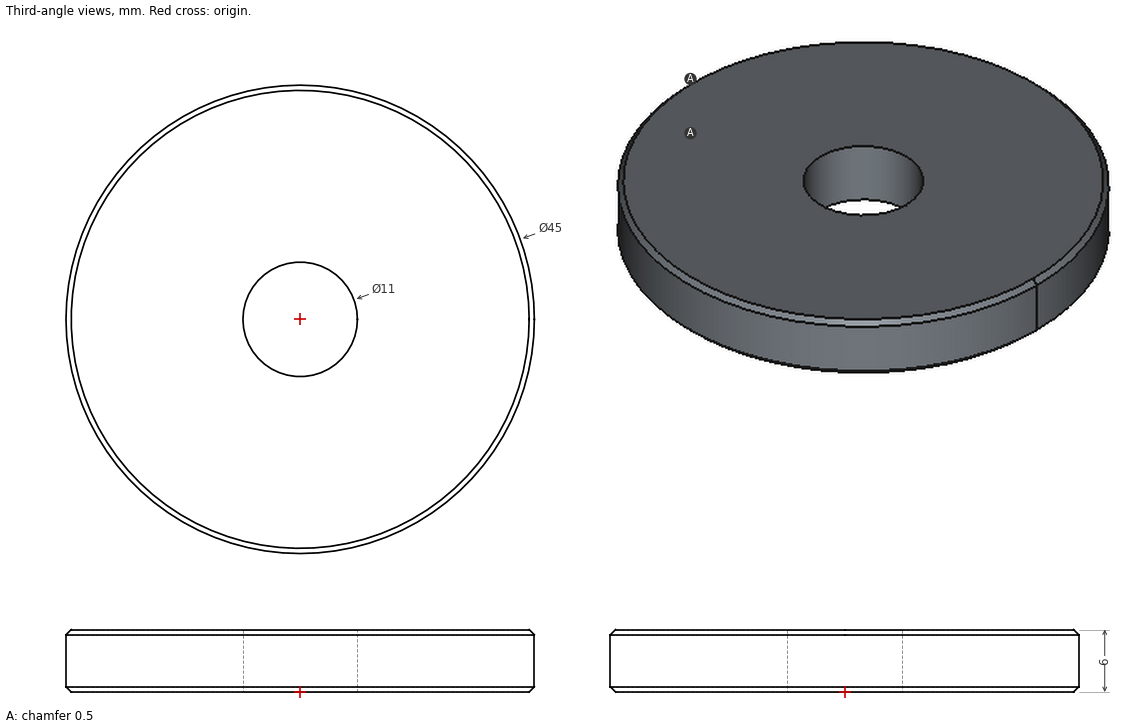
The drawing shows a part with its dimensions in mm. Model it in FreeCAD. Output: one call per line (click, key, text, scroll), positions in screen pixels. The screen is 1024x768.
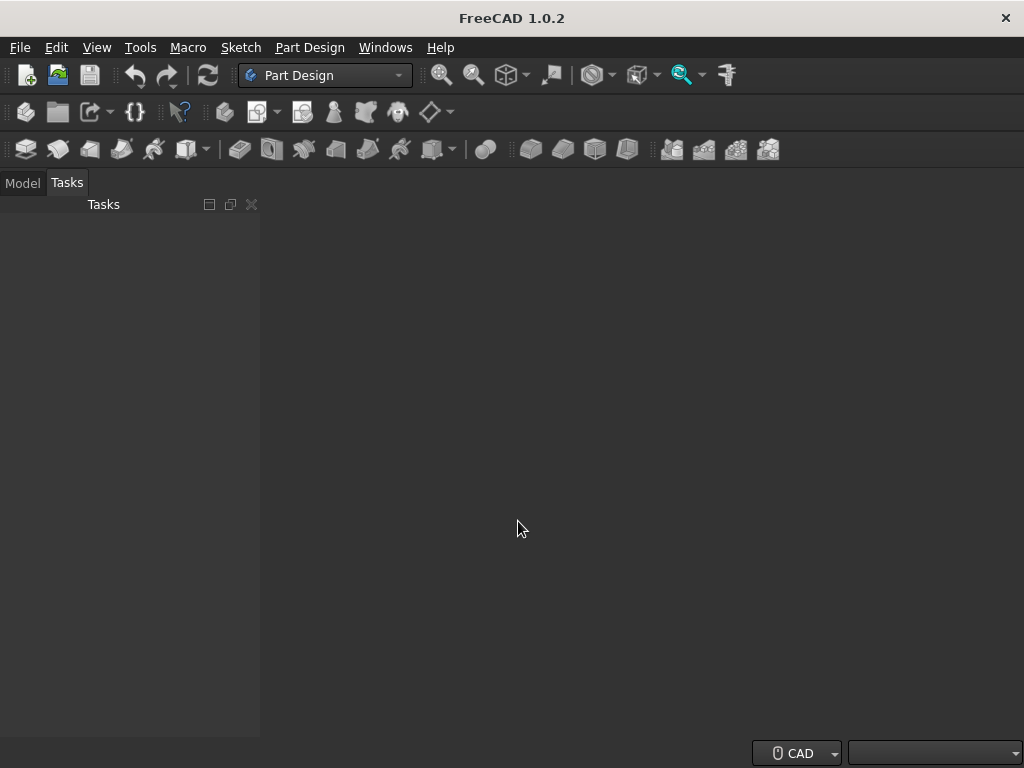
click(26, 76)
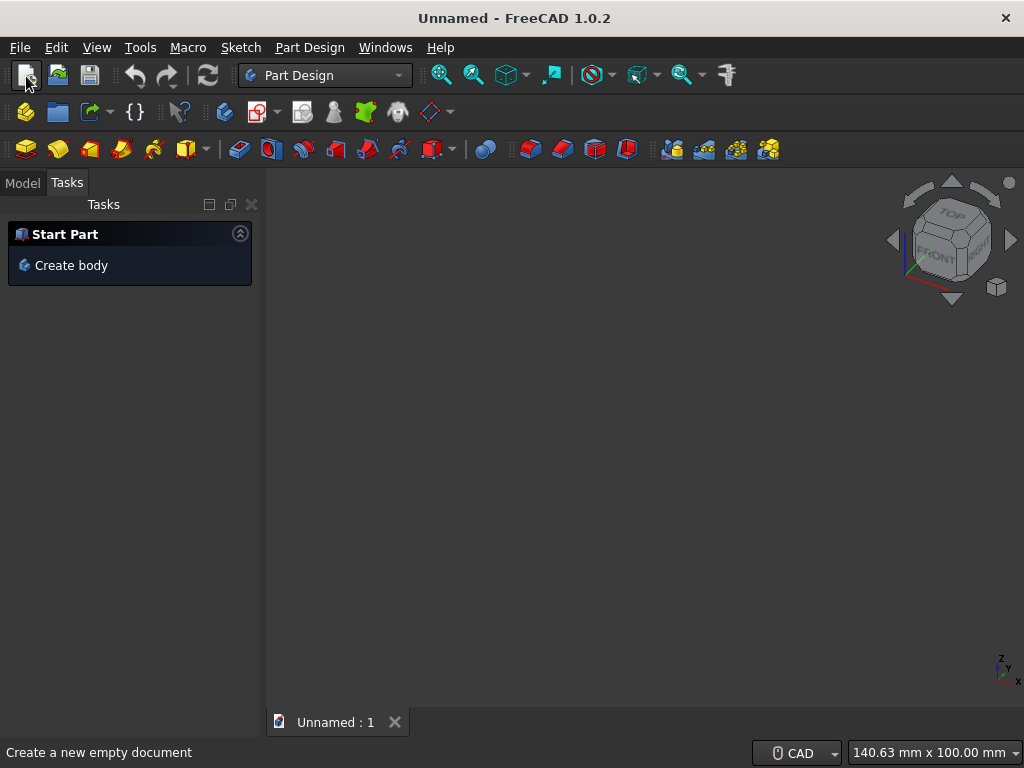
click(258, 112)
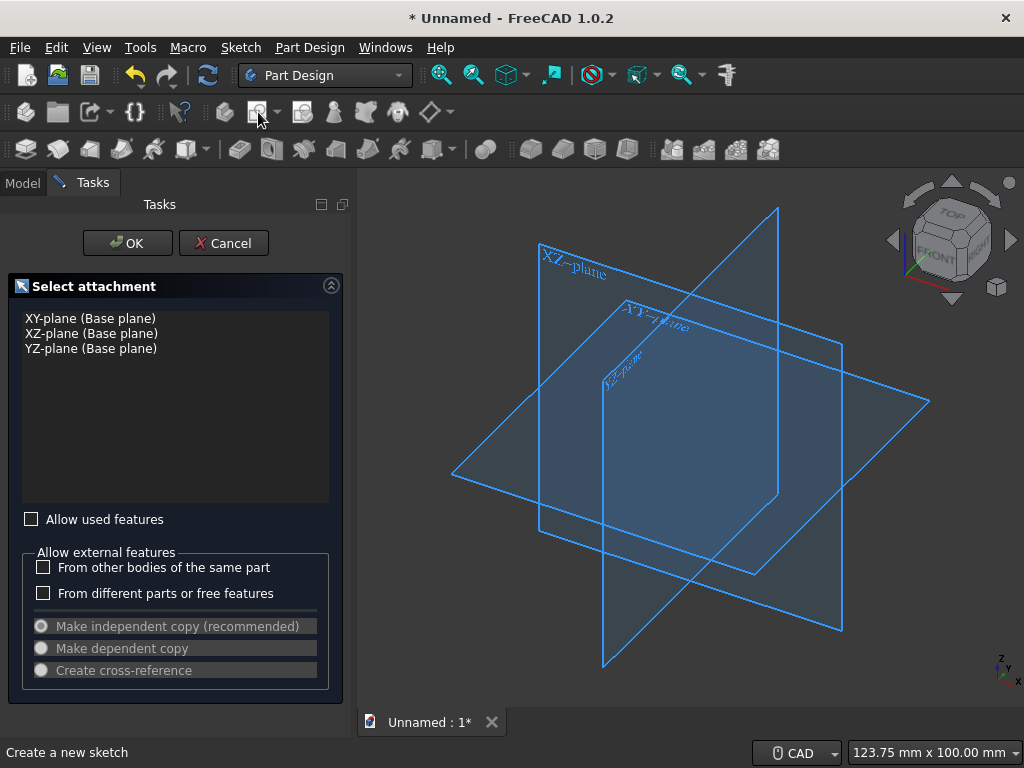
click(82, 318)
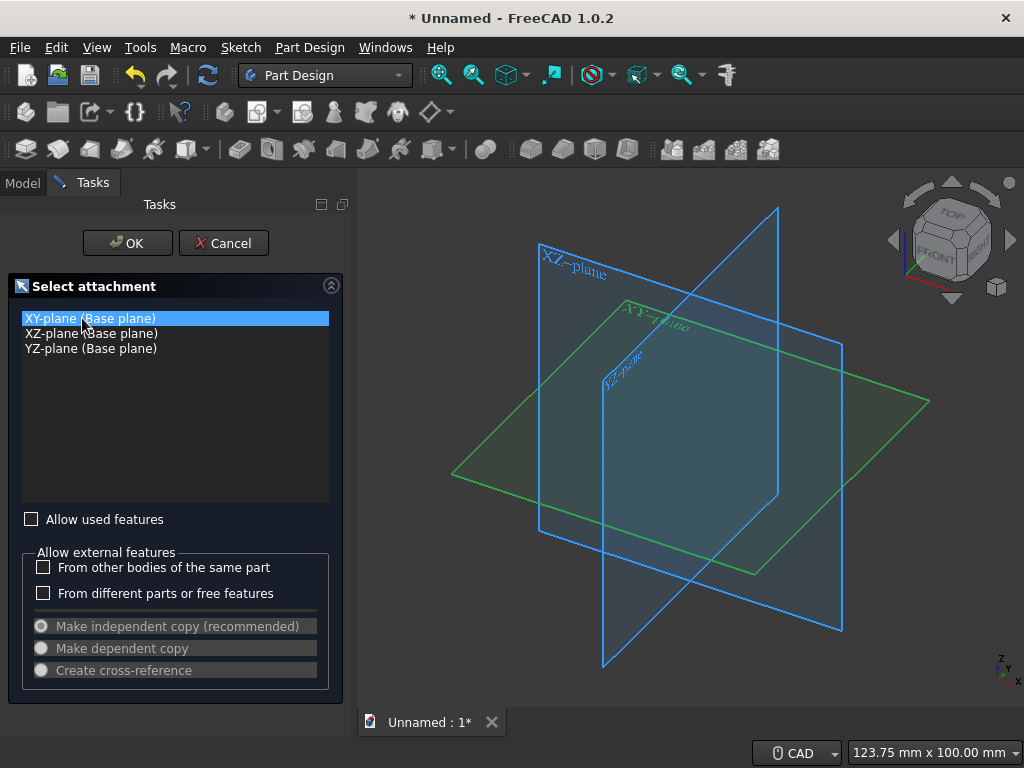
click(128, 243)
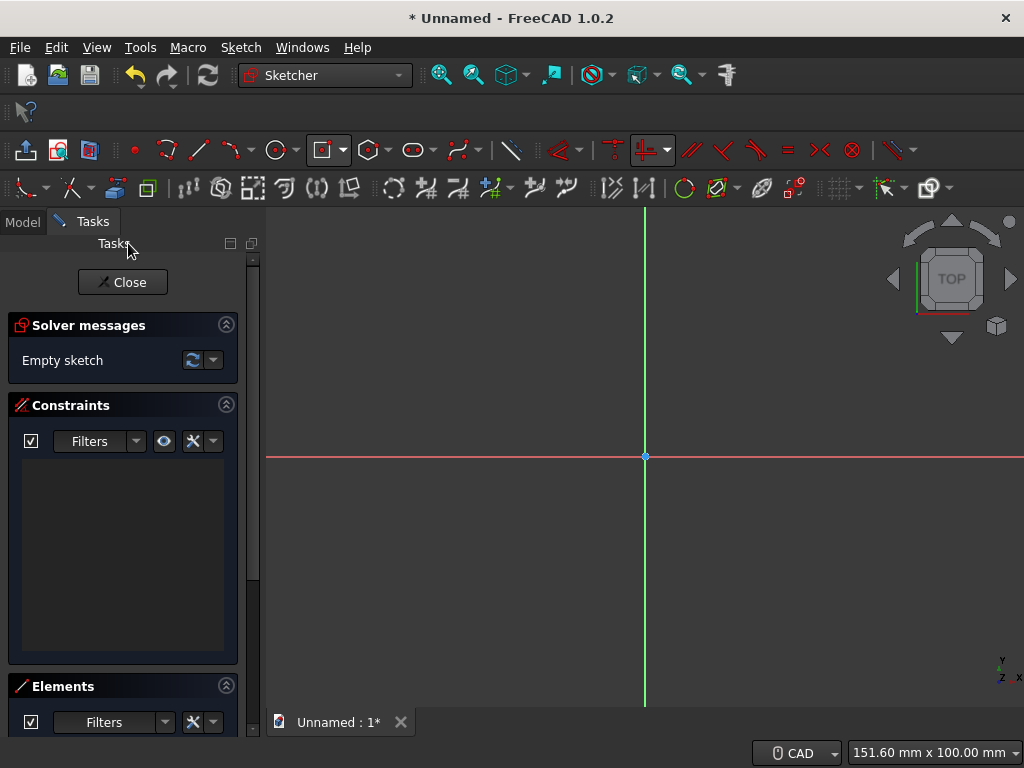
scroll(784, 457, up, 2)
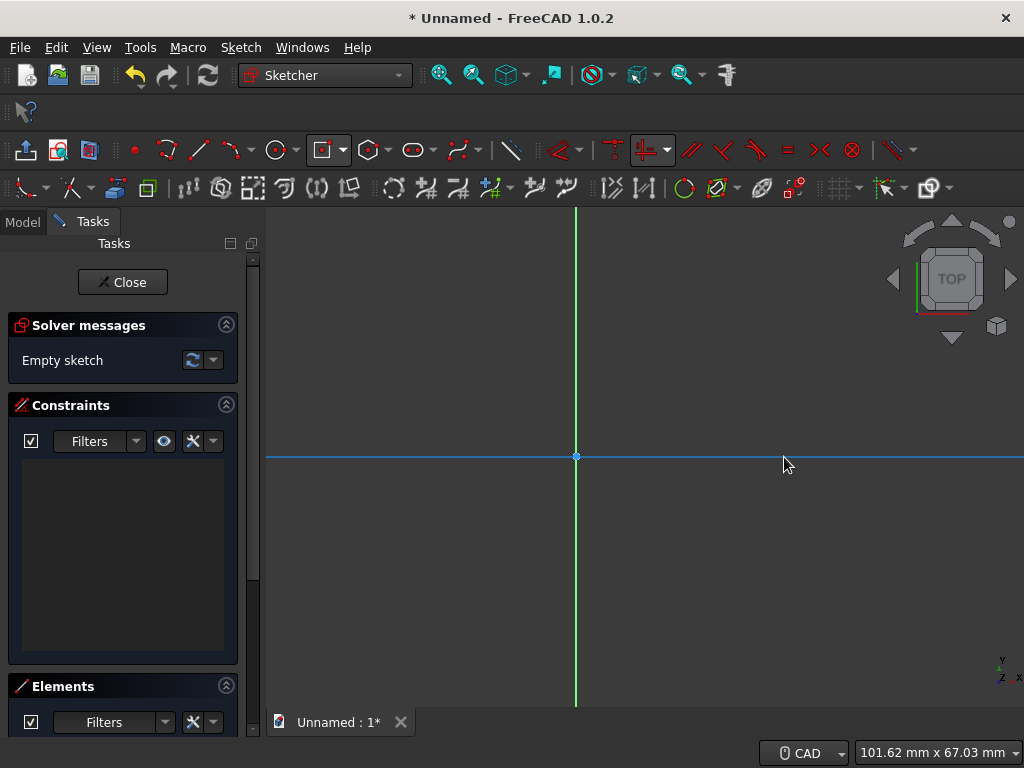
click(276, 150)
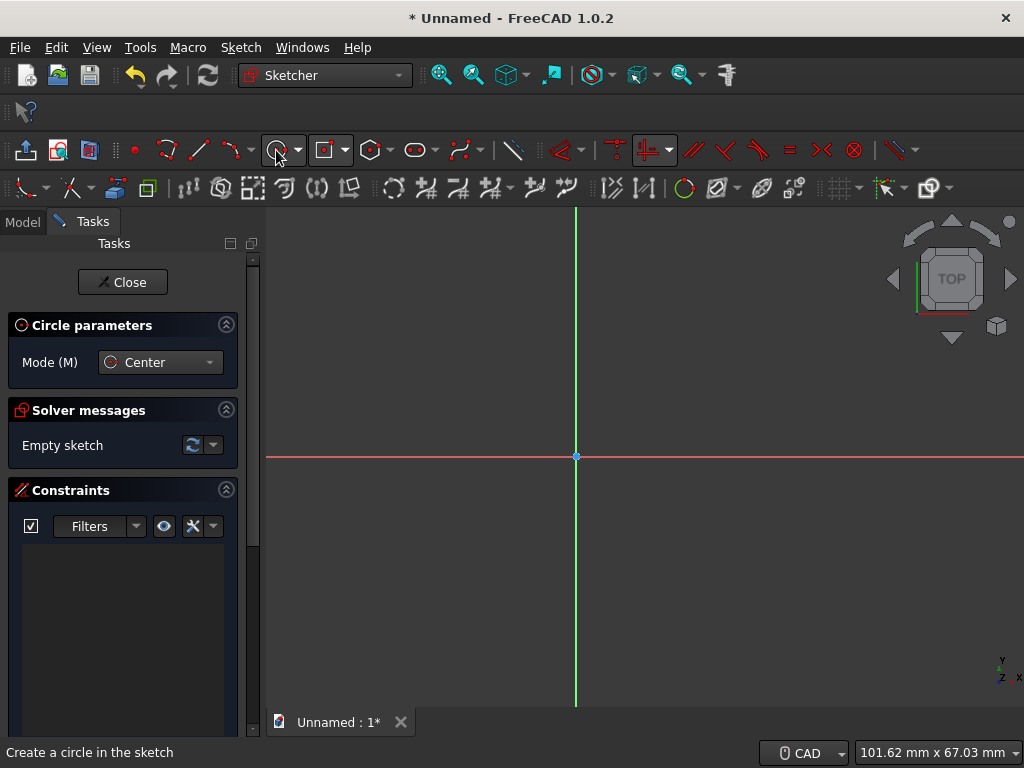
click(576, 457)
move(695, 338)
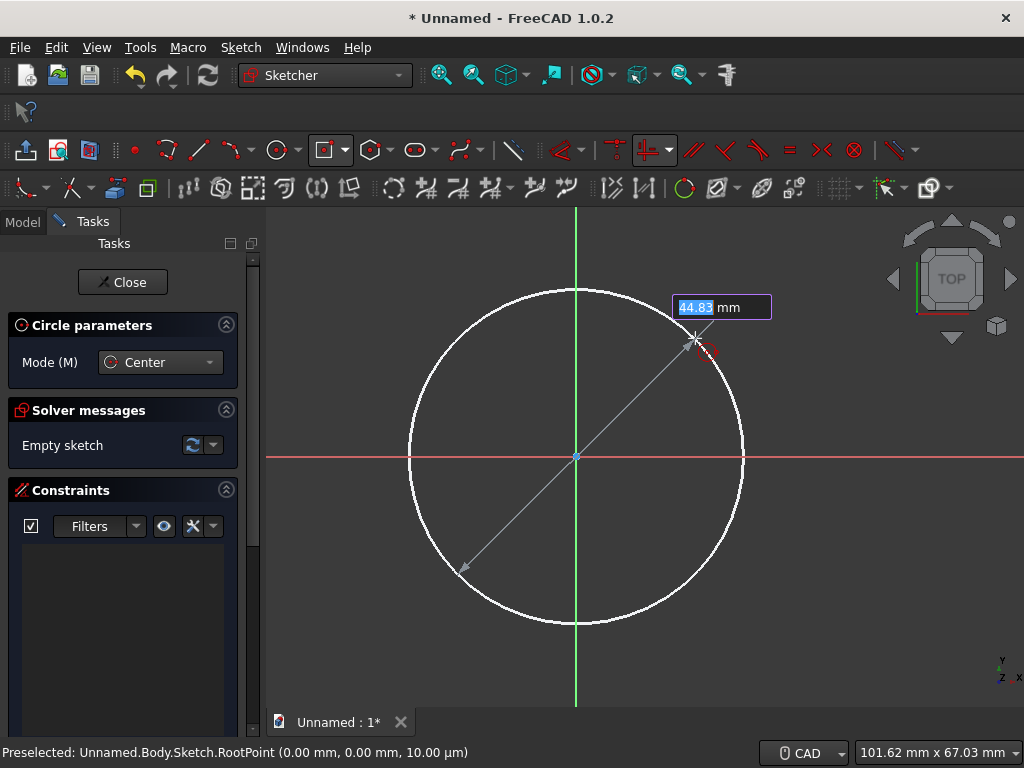
text(45)
key(Return)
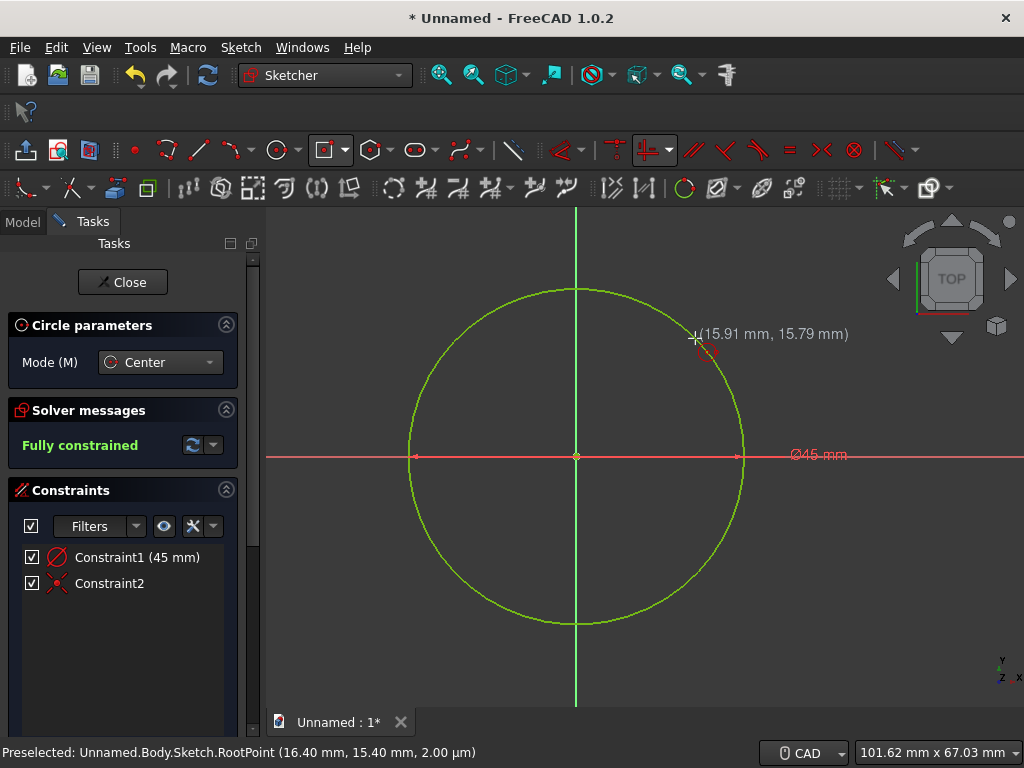
click(576, 457)
move(605, 428)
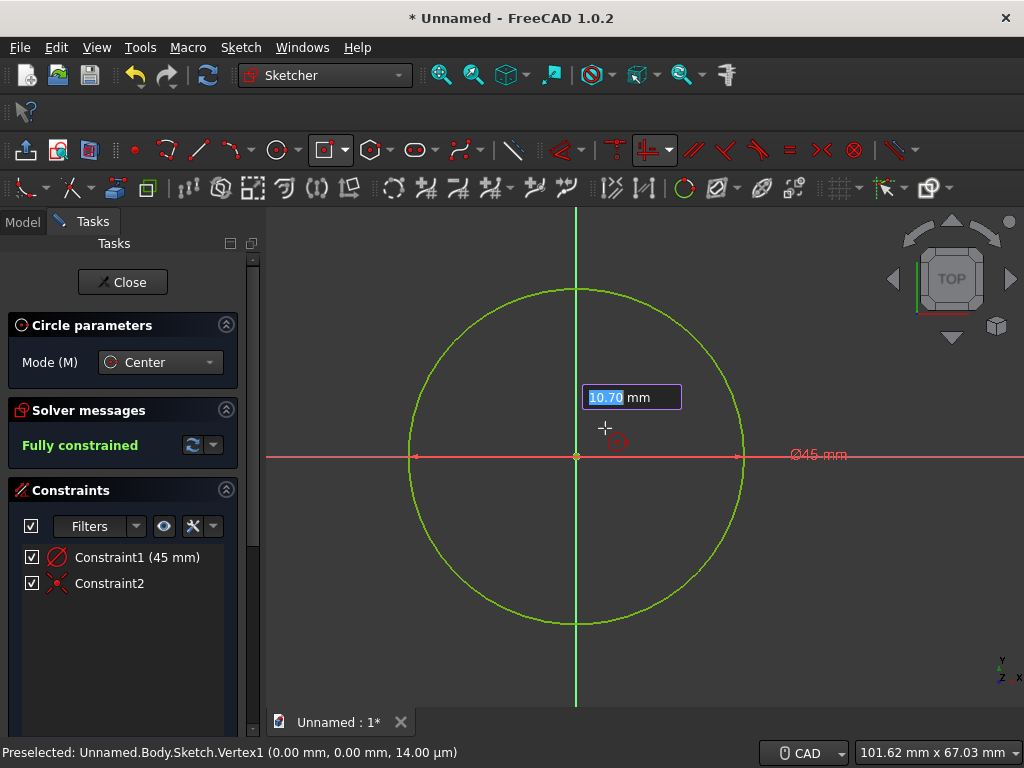
text(11)
key(Return)
key(Escape)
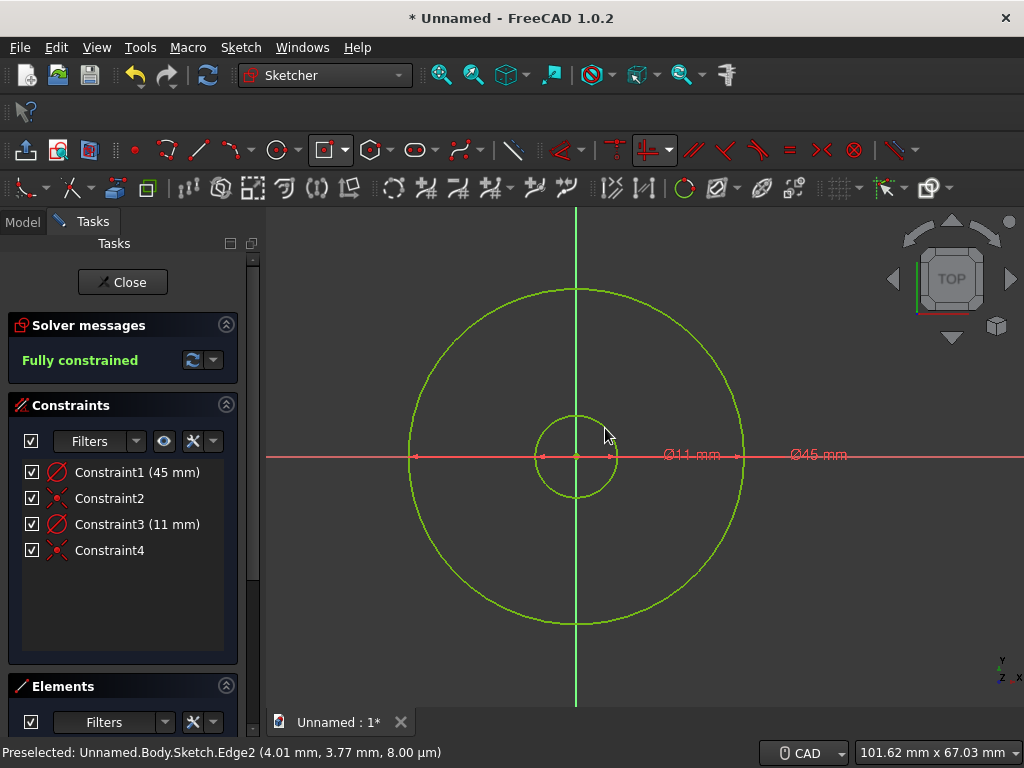
click(123, 282)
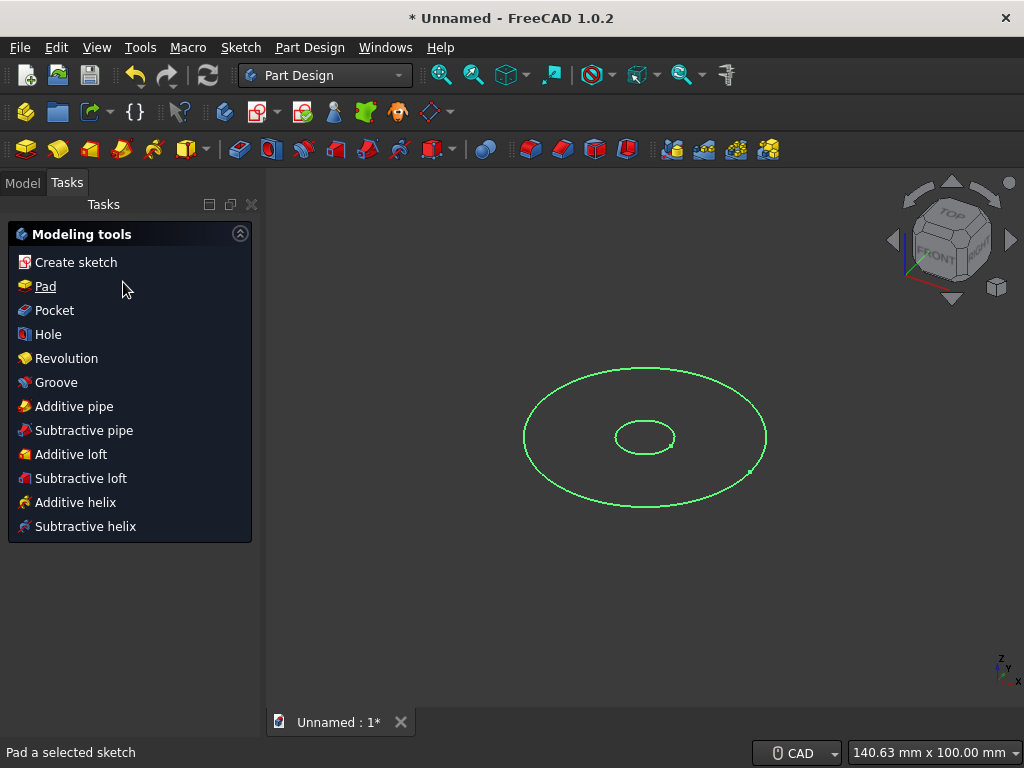
click(26, 150)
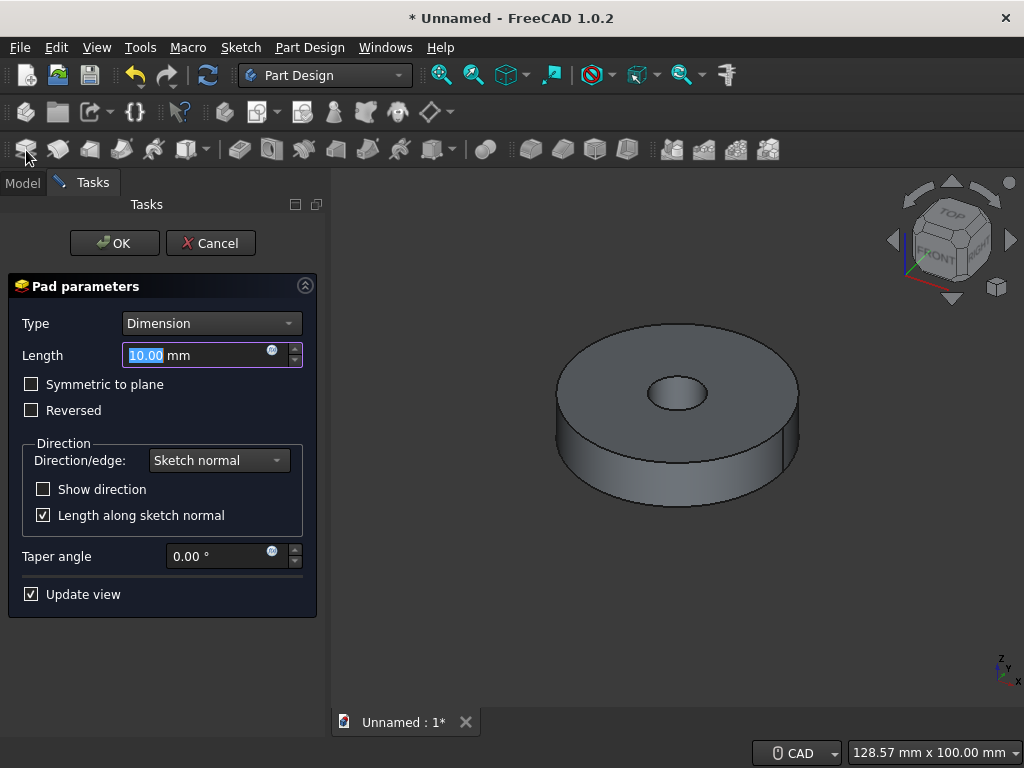
text(6)
key(Tab)